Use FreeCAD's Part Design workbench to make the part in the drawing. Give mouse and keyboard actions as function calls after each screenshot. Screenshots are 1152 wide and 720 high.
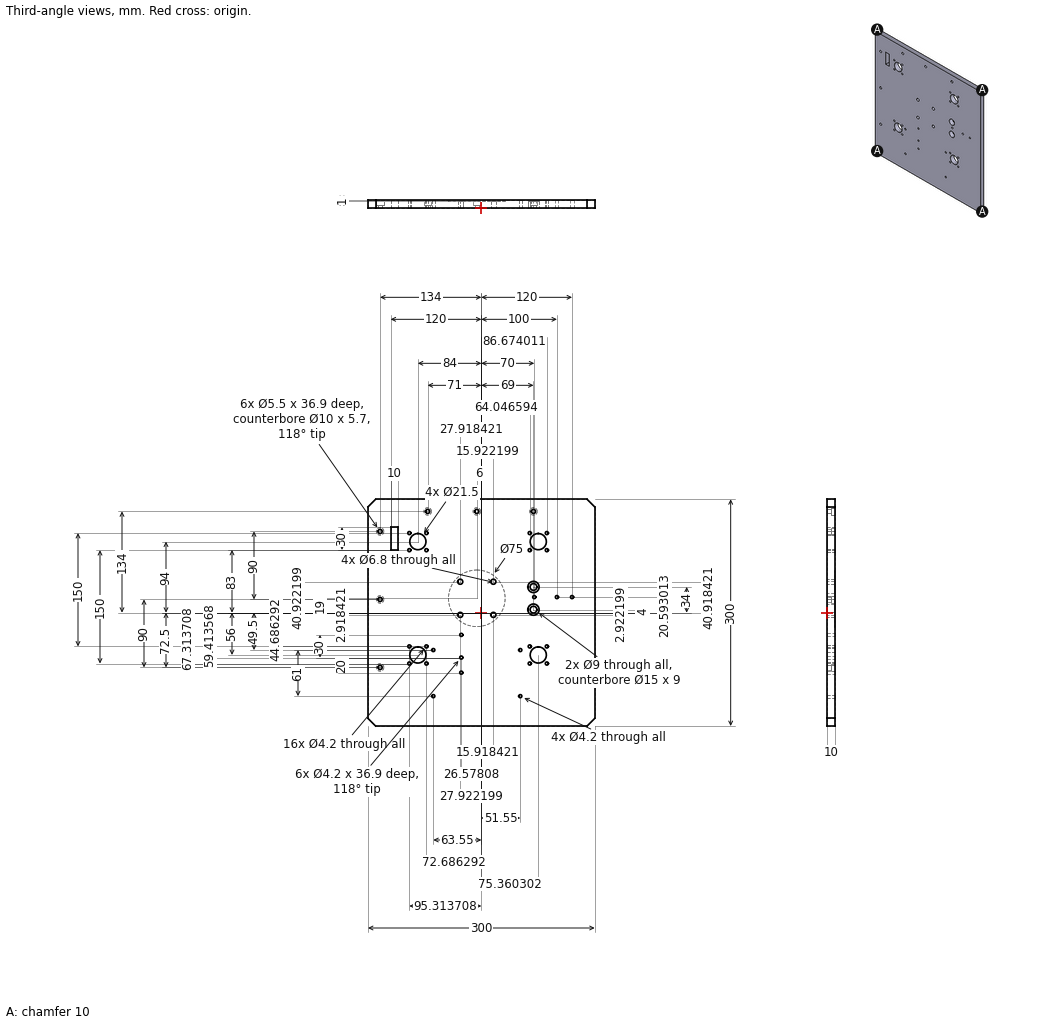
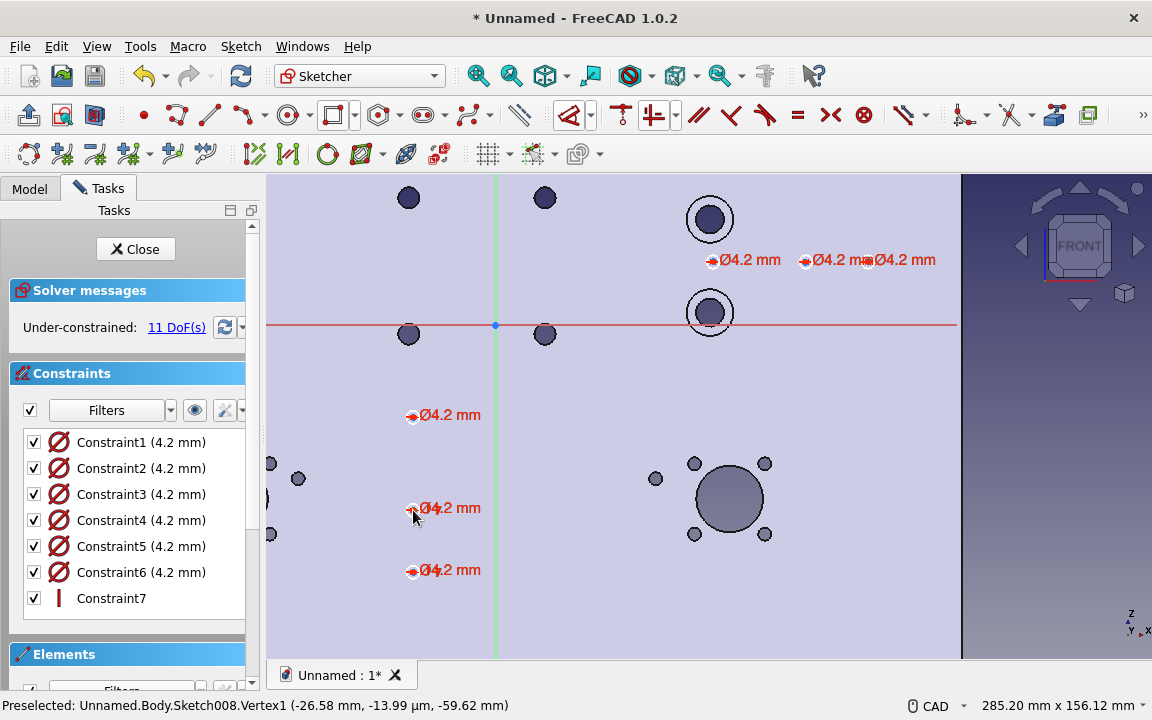
click(413, 417)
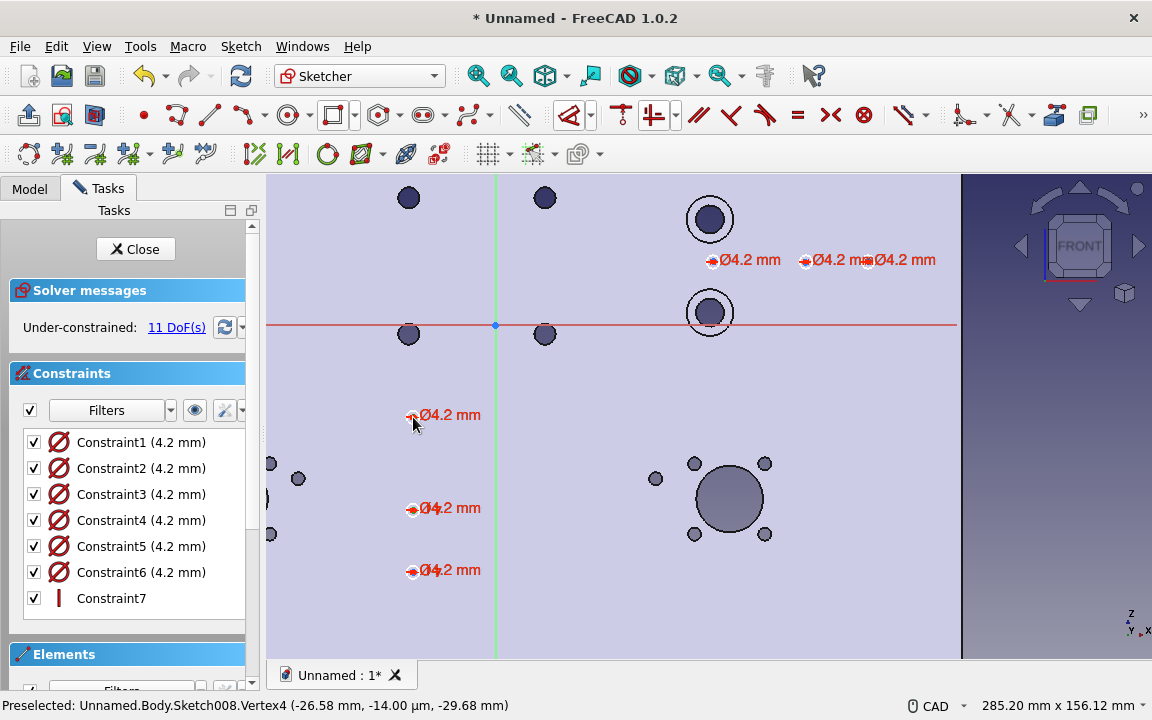
key(v)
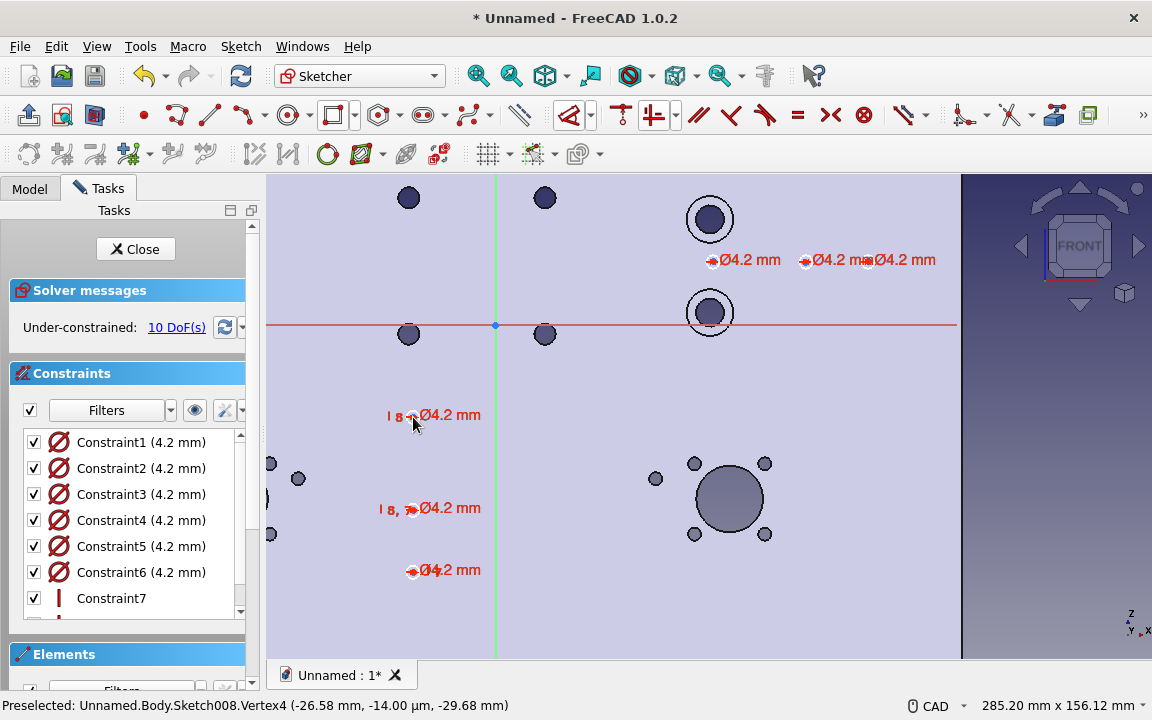
click(806, 262)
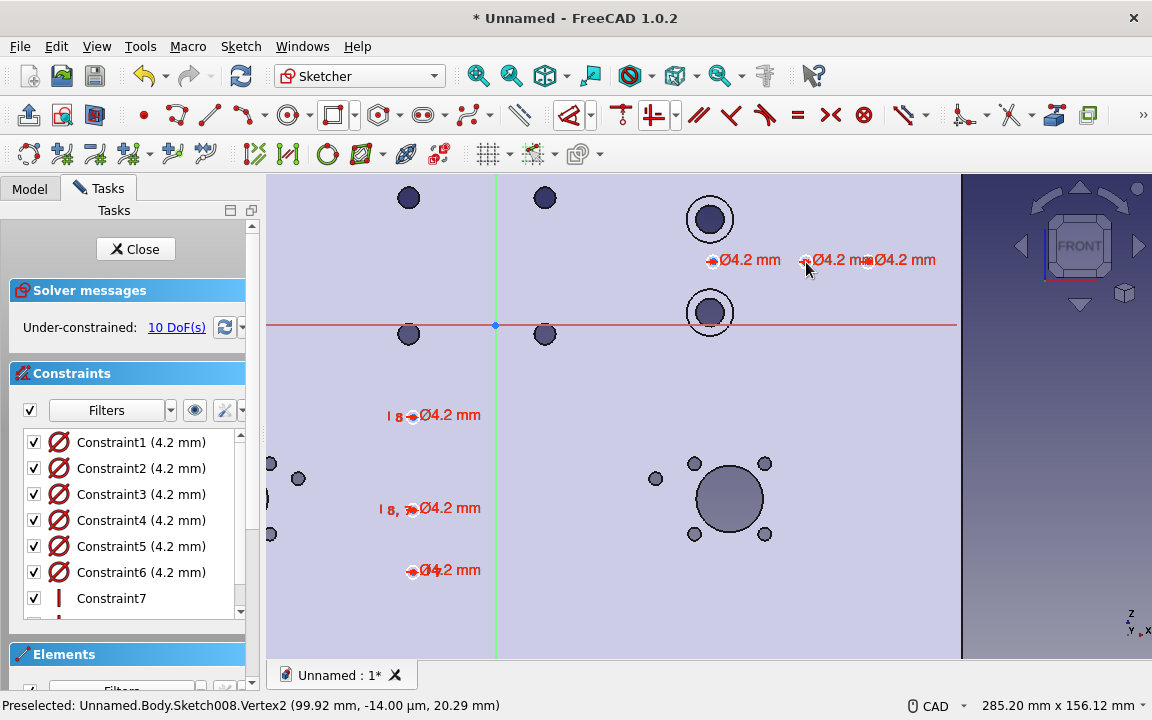
click(868, 262)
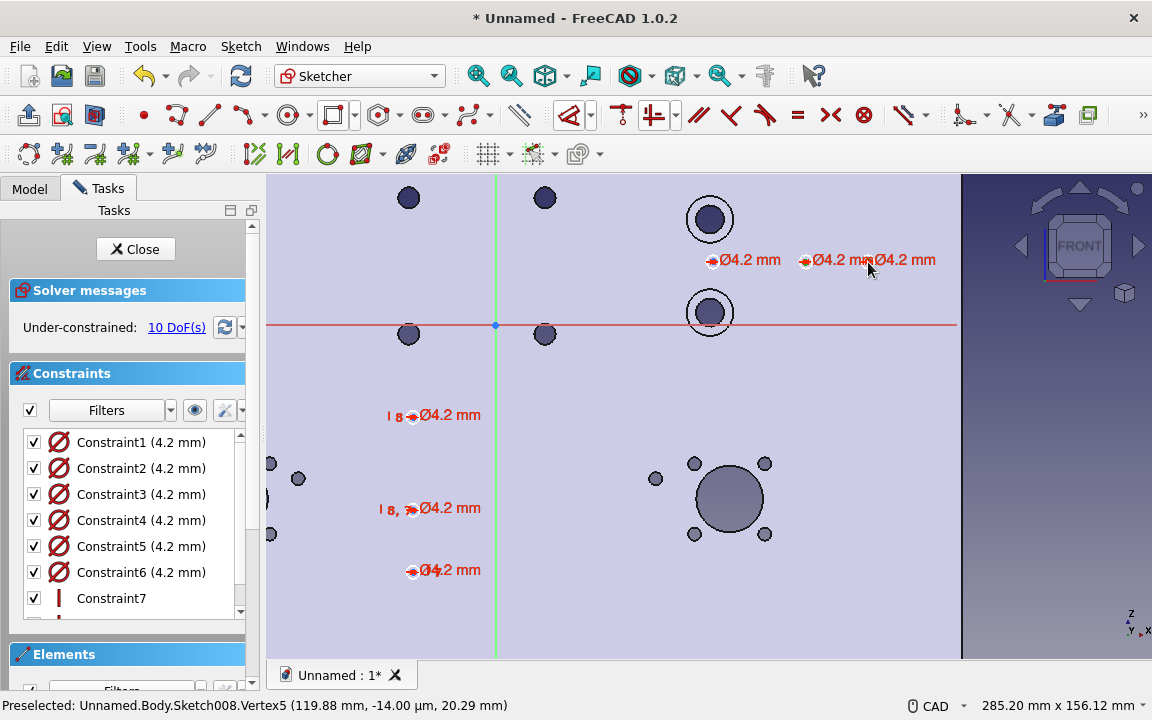
click(676, 116)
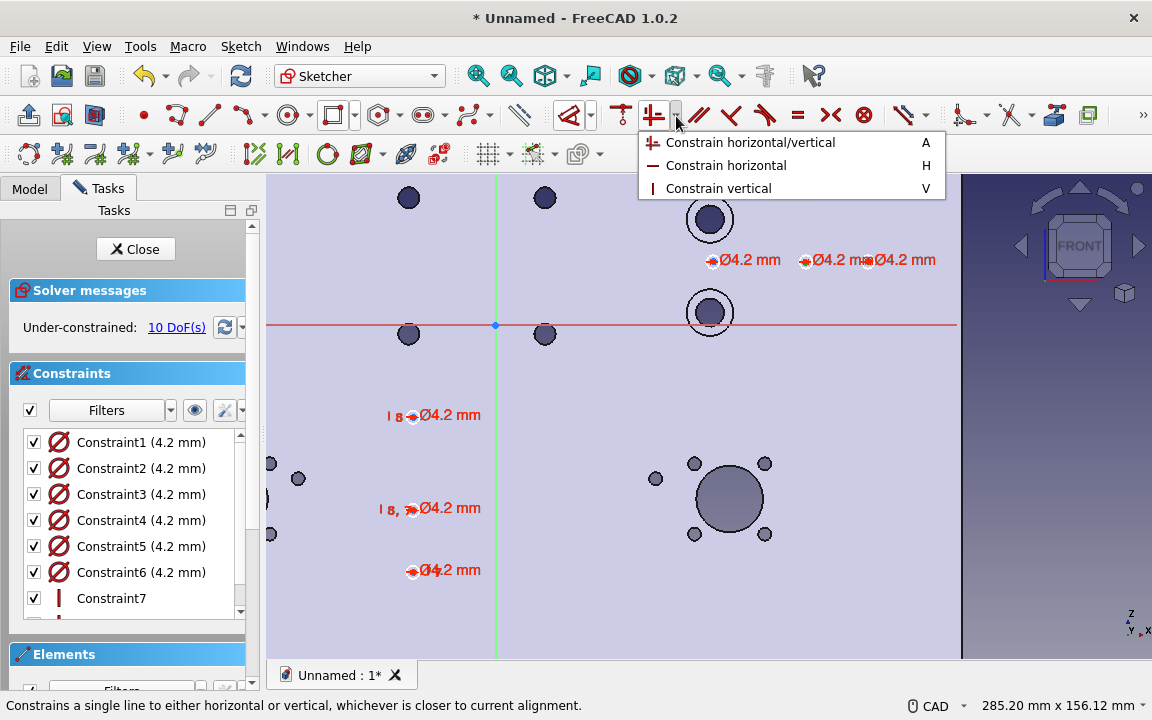
click(792, 166)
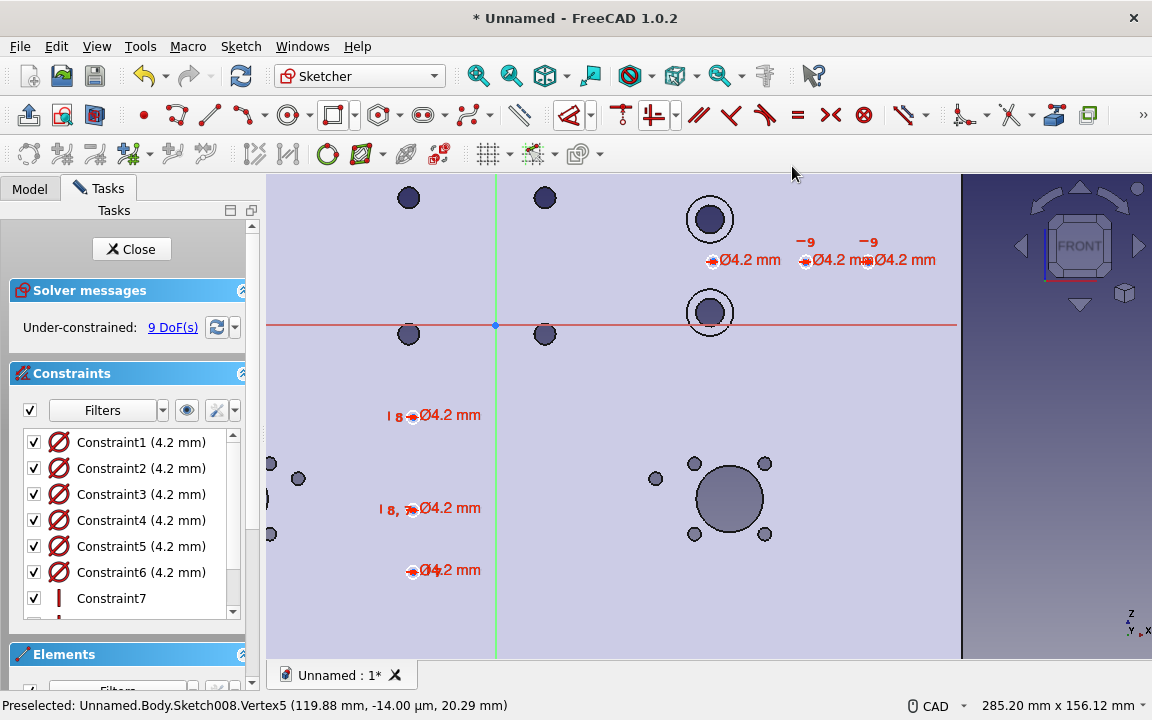
click(806, 262)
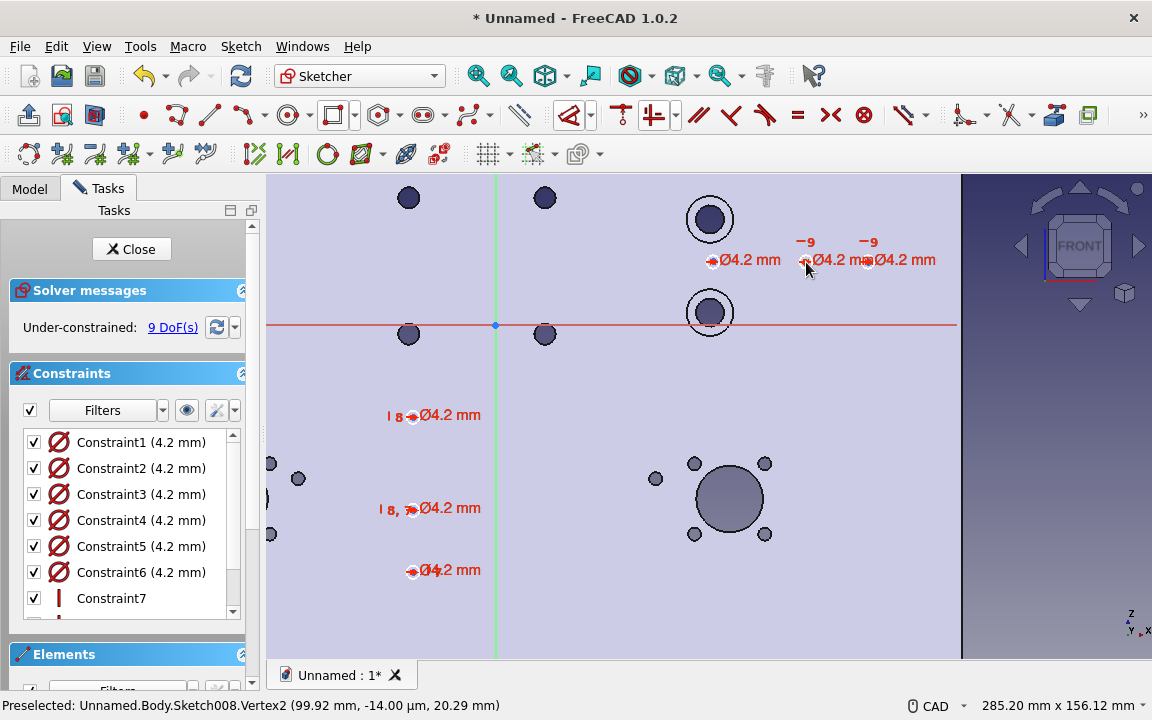
click(713, 262)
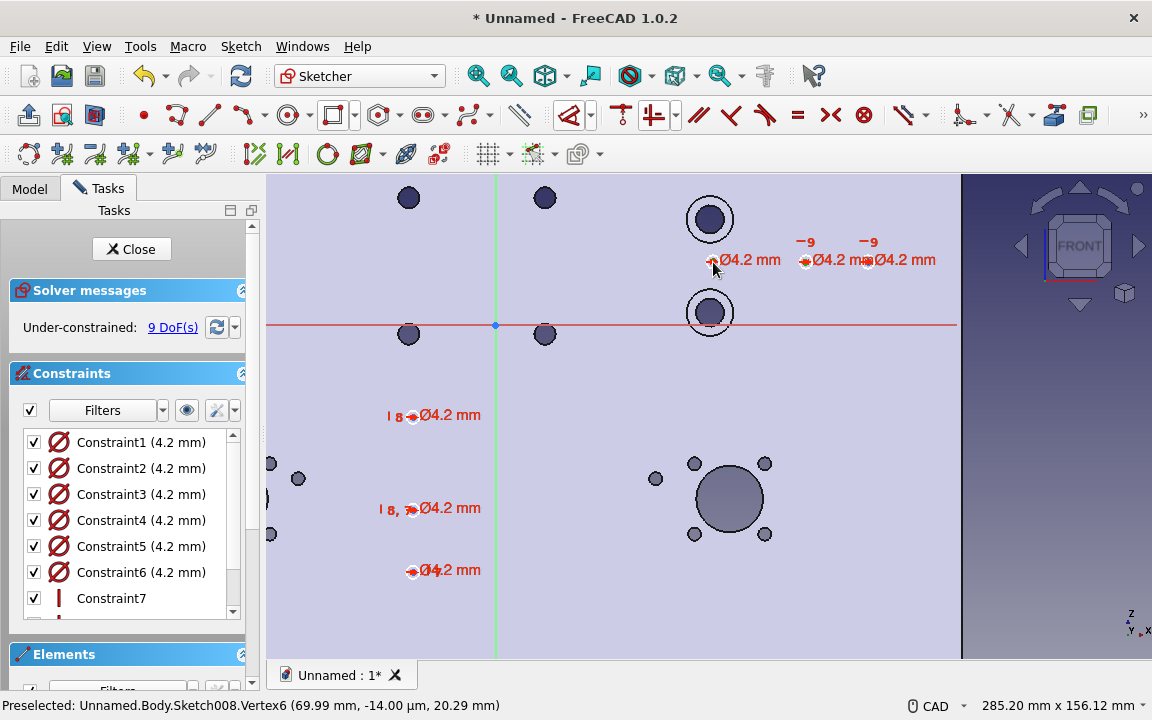
key(h)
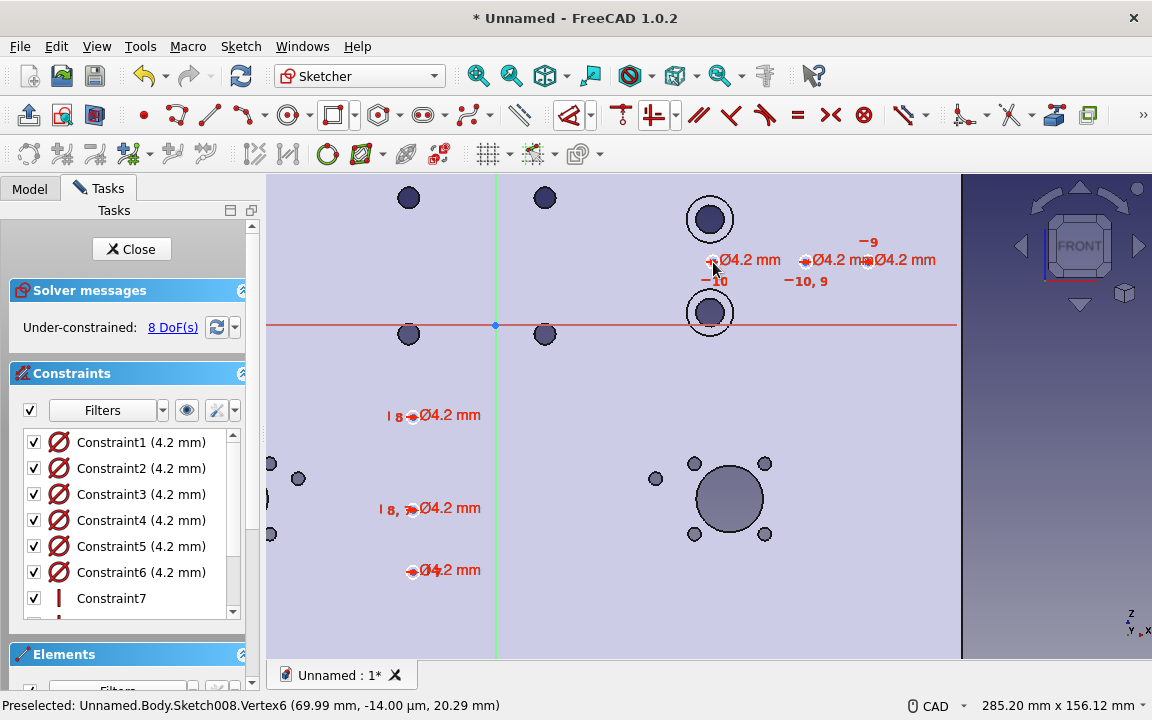
click(713, 262)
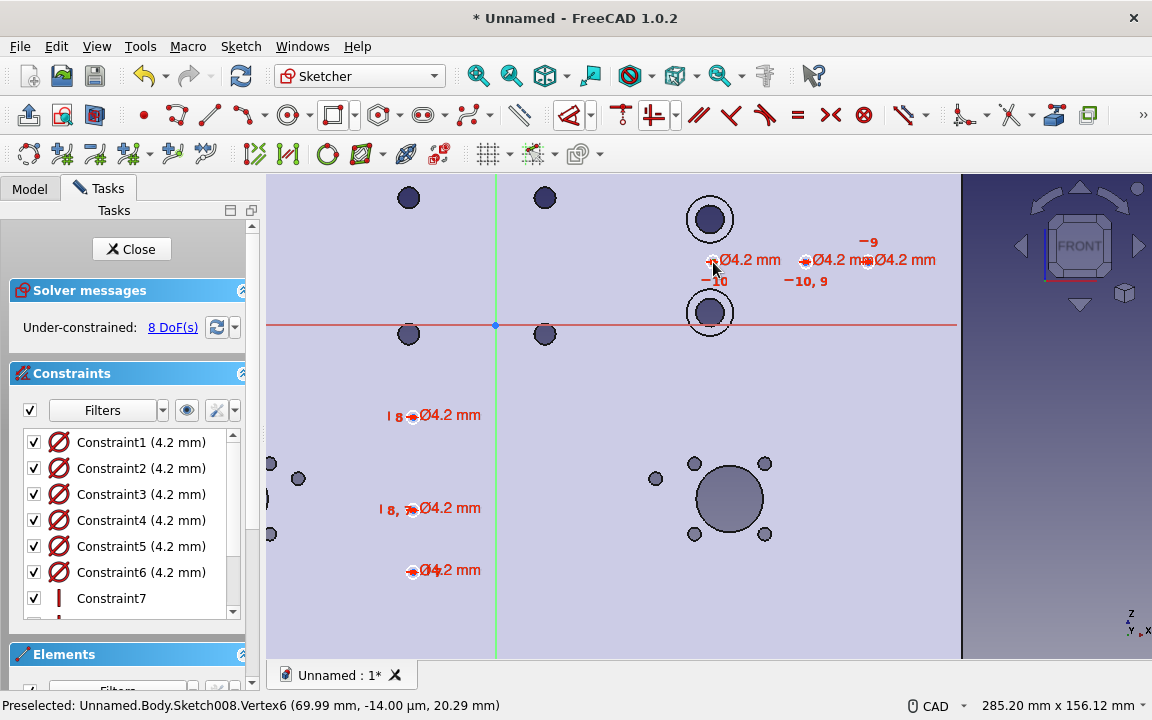
key(l)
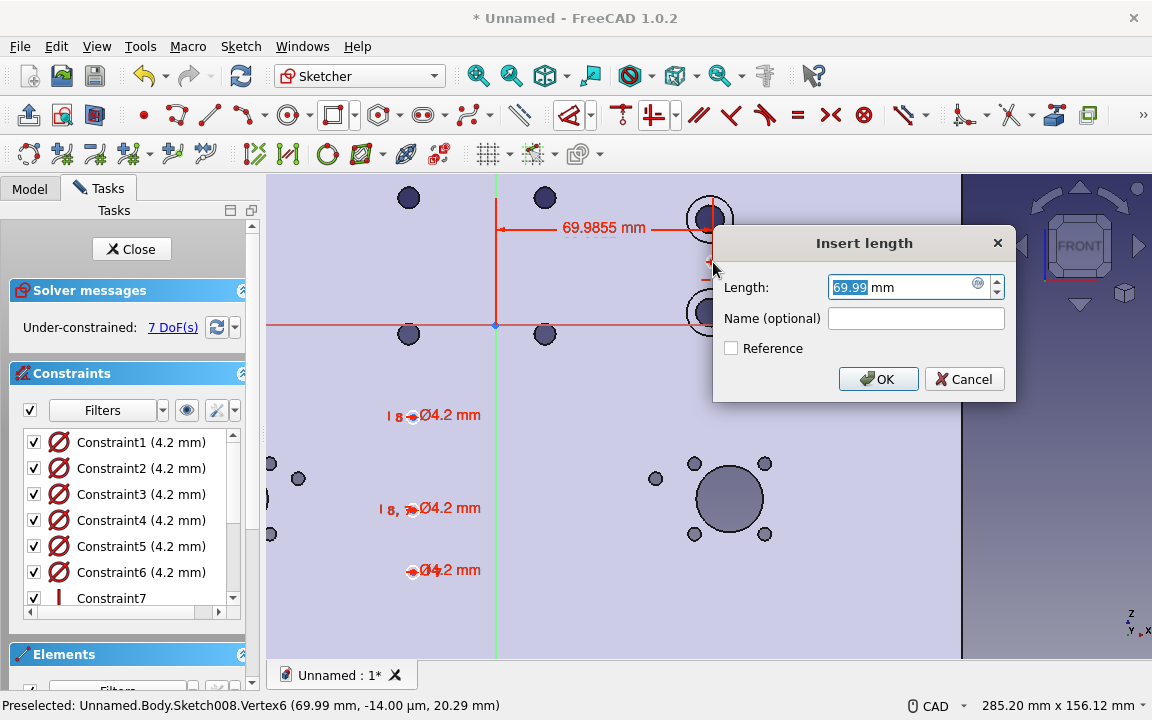
text(70)
key(Return)